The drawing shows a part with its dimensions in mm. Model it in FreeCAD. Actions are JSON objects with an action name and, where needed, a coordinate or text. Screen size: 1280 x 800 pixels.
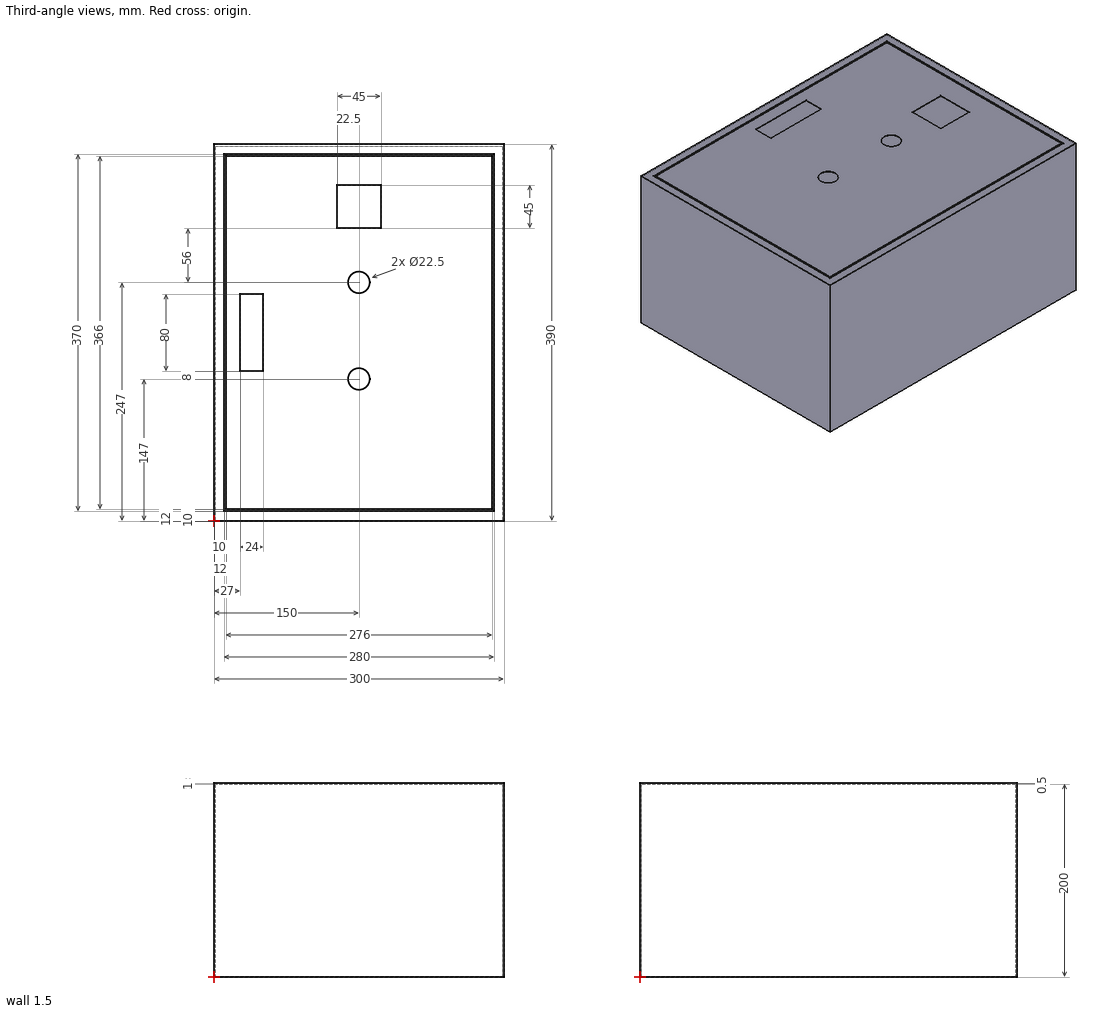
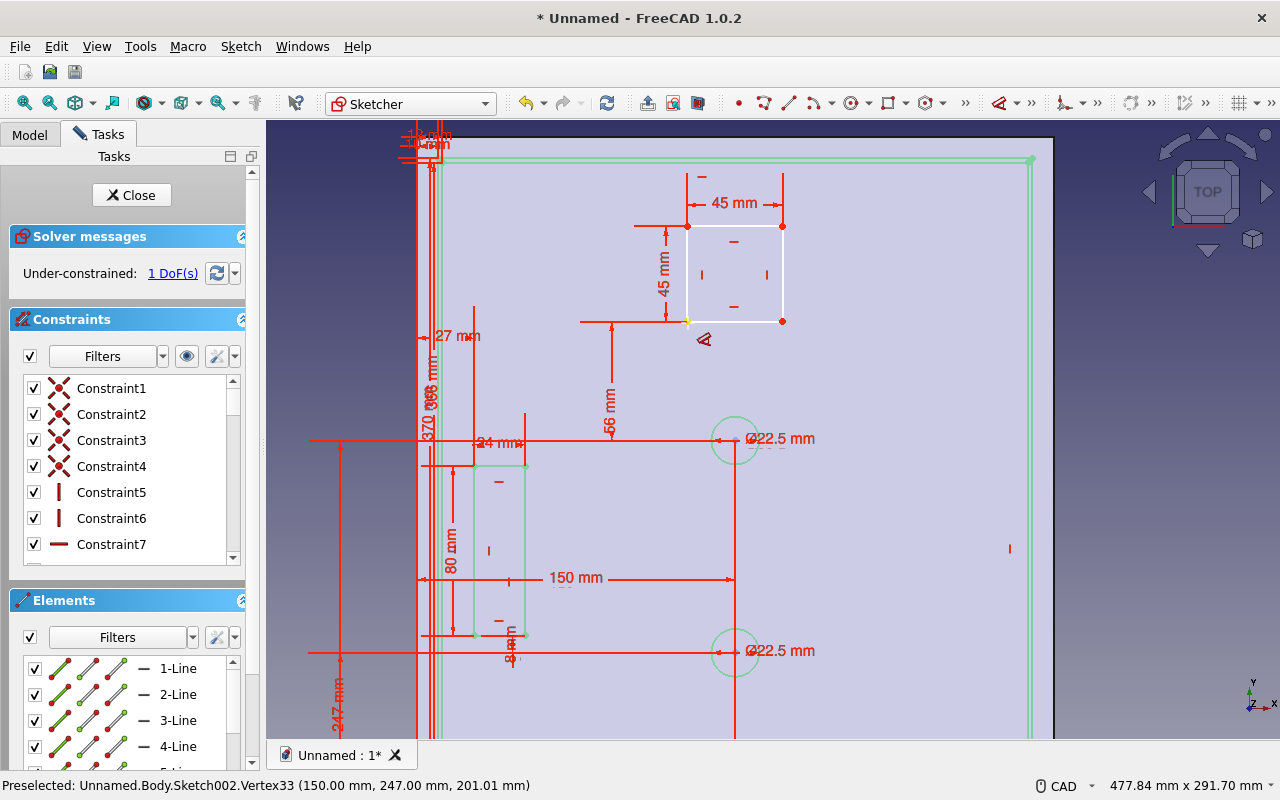
{"action": "left_click", "coordinate": [687, 322]}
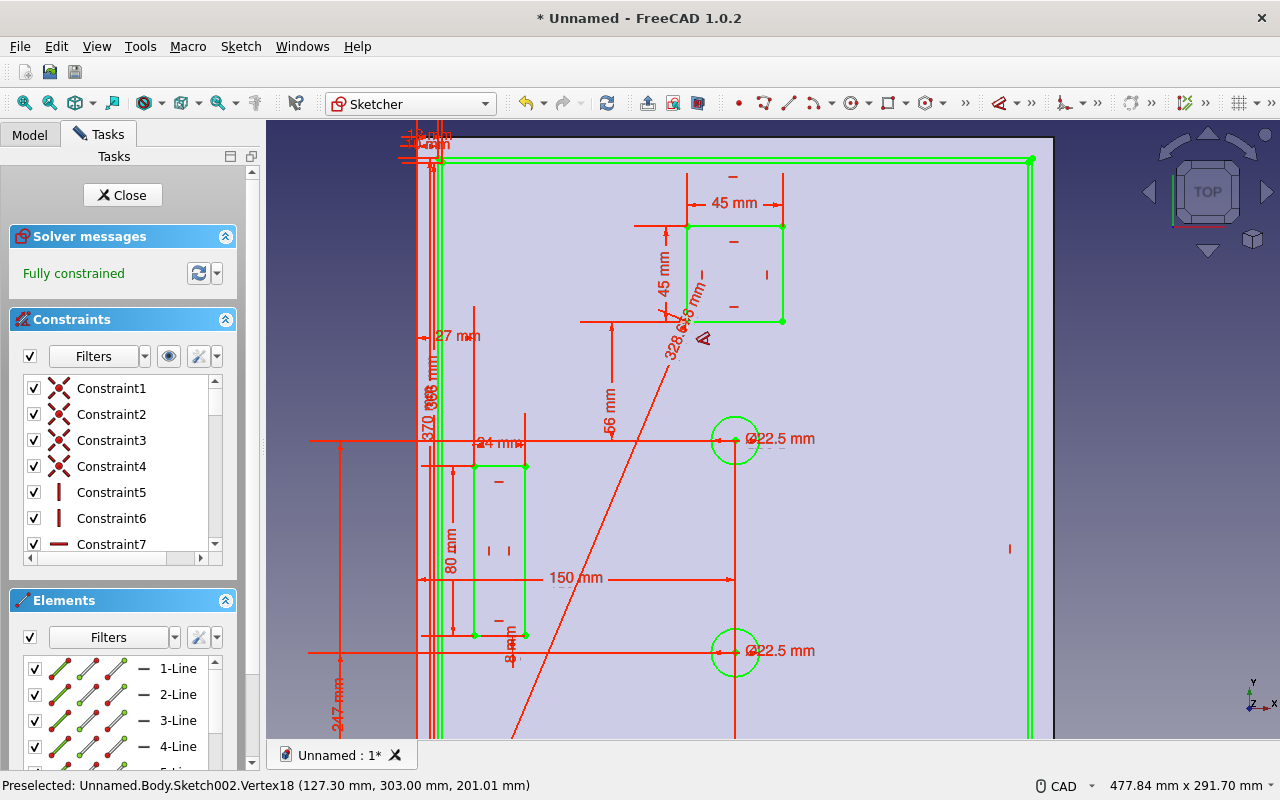
{"action": "left_click", "coordinate": [735, 441]}
{"action": "left_click", "coordinate": [711, 288]}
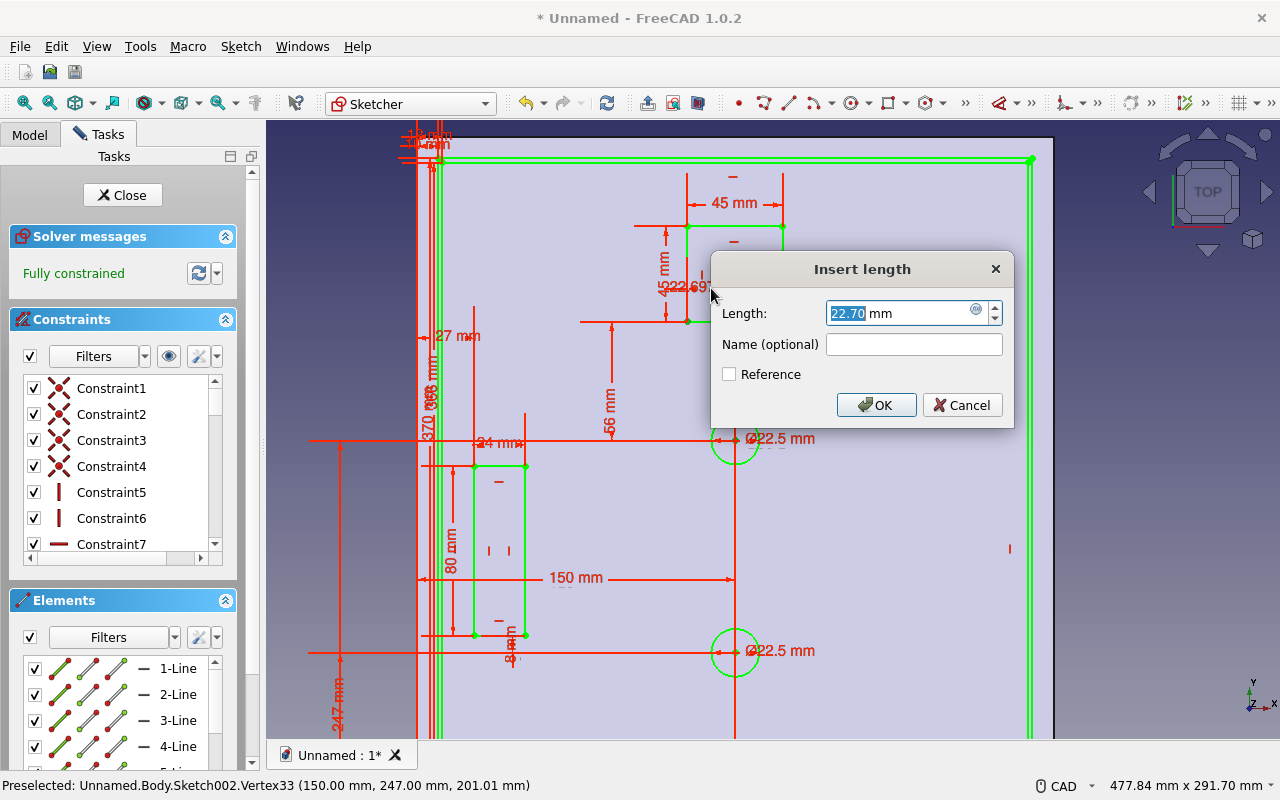
{"action": "type", "text": "22.5"}
{"action": "key", "text": "Return"}
{"action": "key", "text": "Escape"}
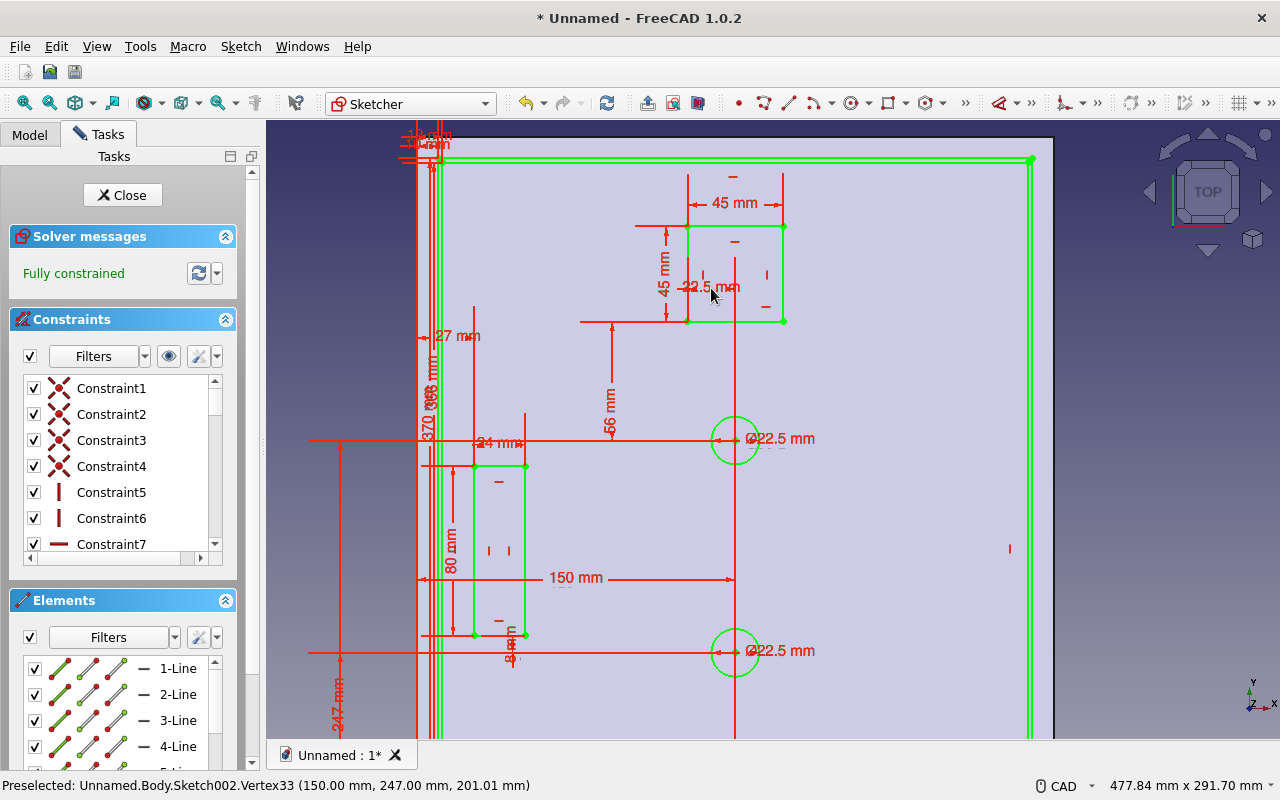
{"action": "left_click", "coordinate": [123, 195]}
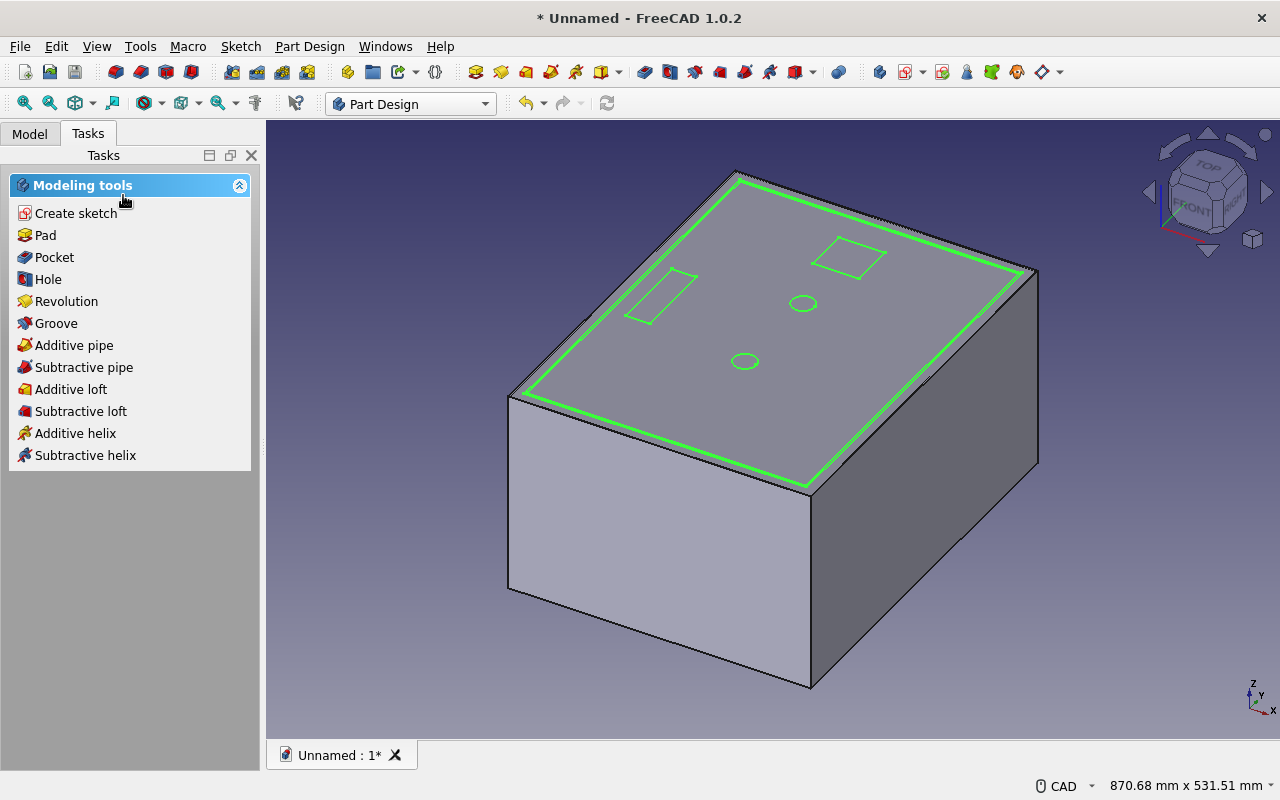
{"action": "left_click", "coordinate": [645, 72]}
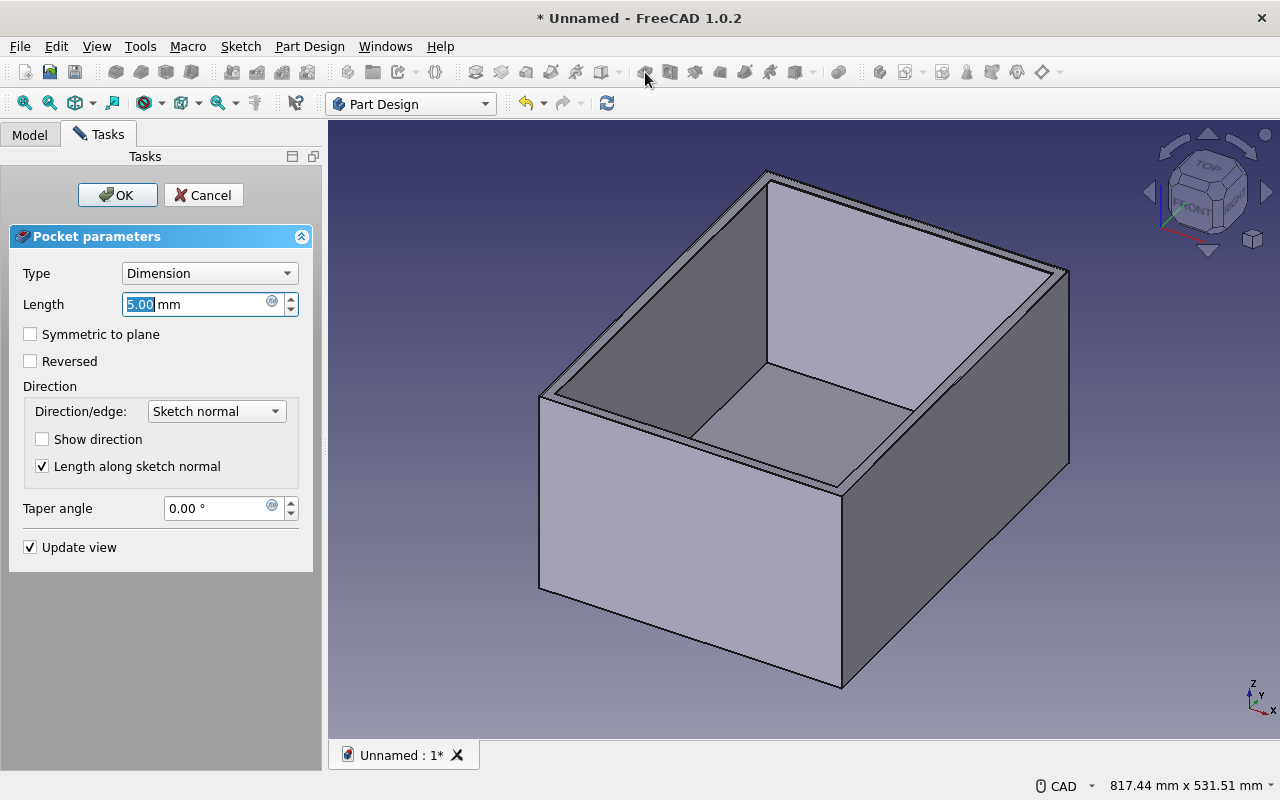
{"action": "type", "text": "0.5"}
{"action": "key", "text": "Tab"}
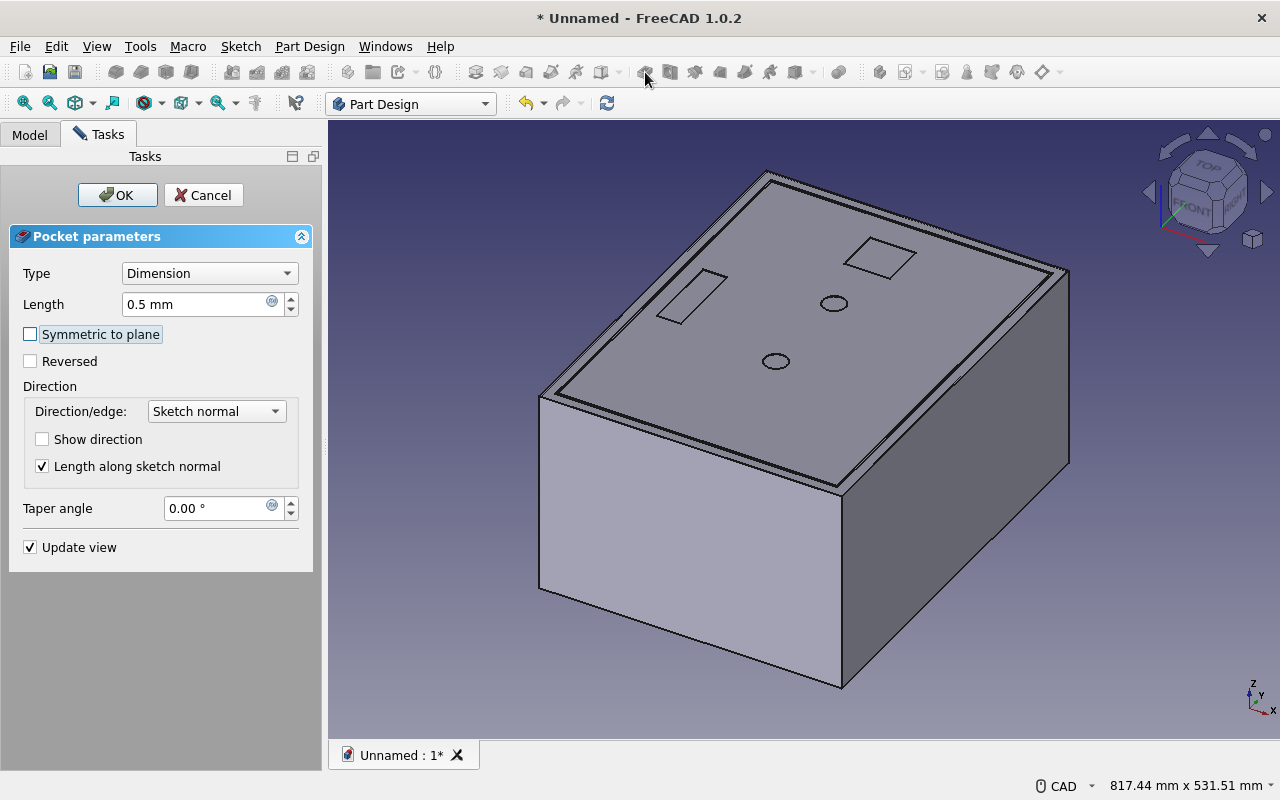
{"action": "left_click", "coordinate": [118, 195]}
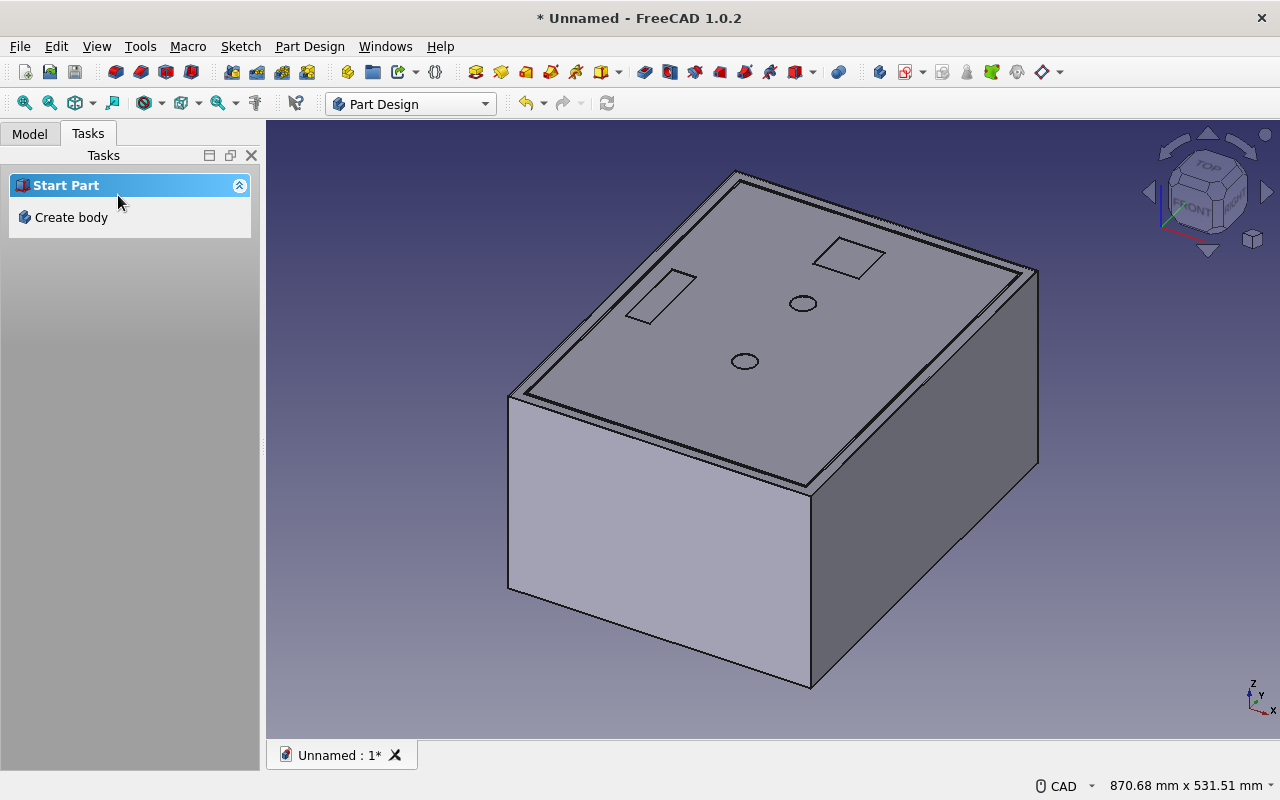
{"action": "key", "text": "0"}